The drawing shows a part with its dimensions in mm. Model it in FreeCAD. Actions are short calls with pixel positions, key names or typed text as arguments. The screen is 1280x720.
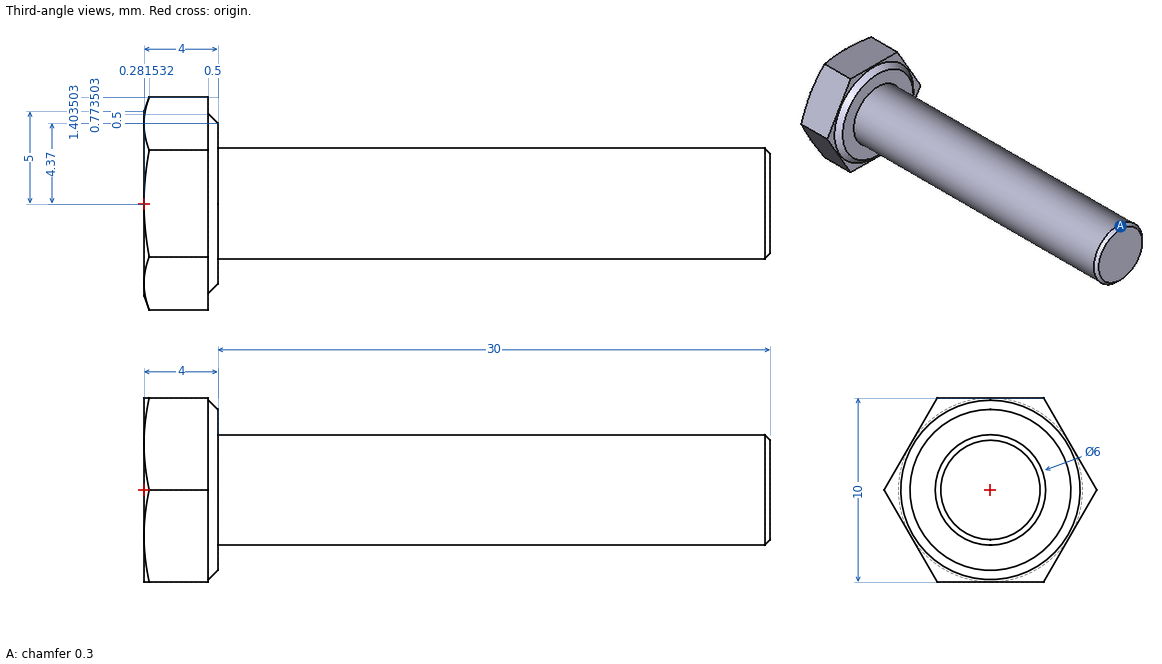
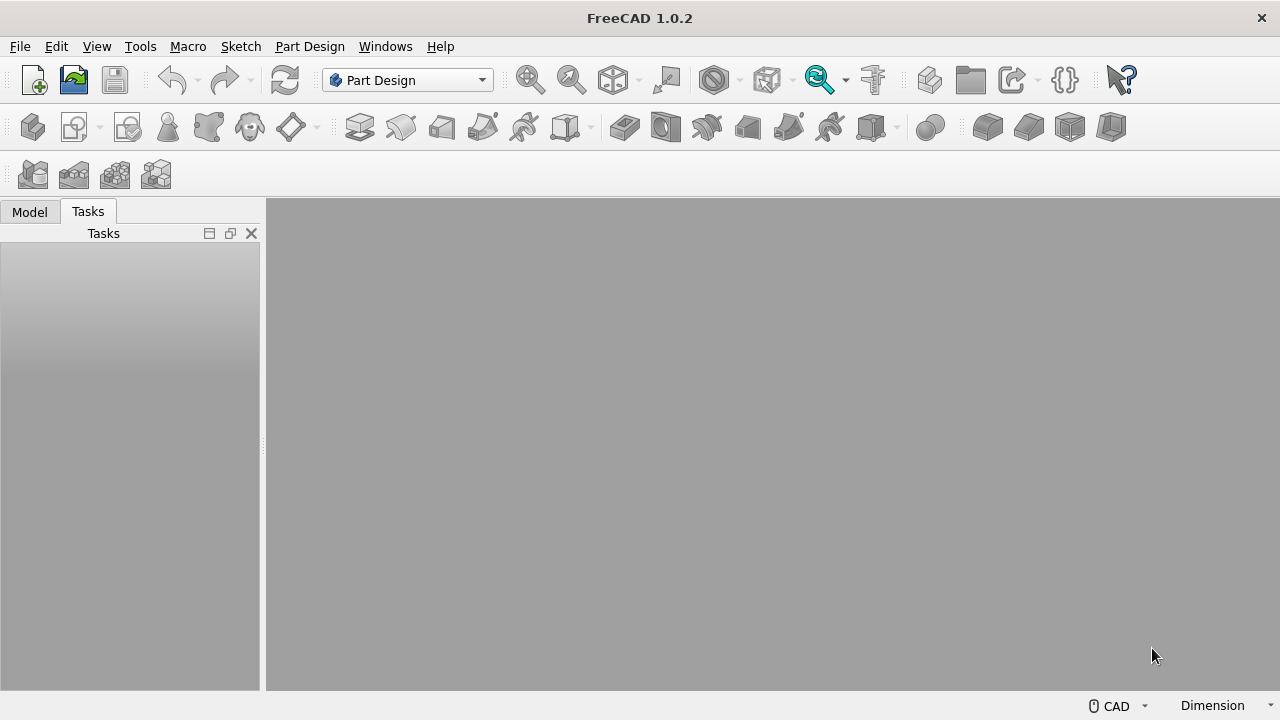
click(33, 80)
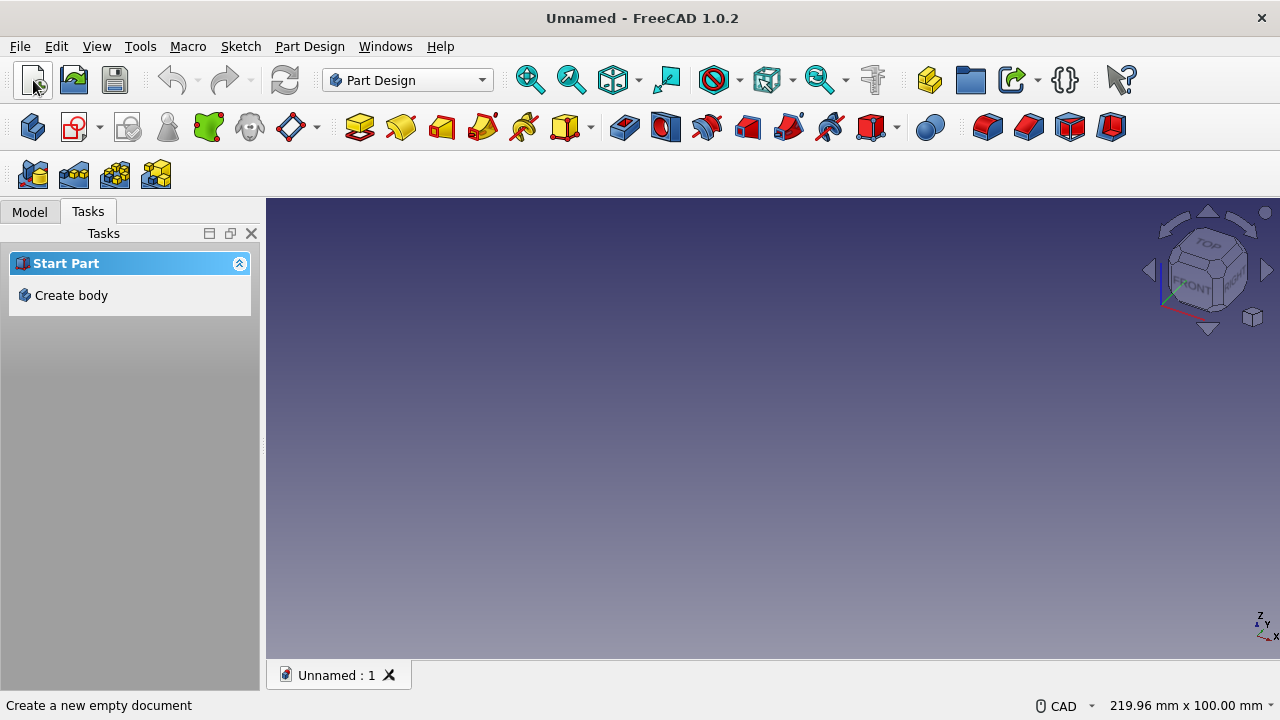
click(74, 128)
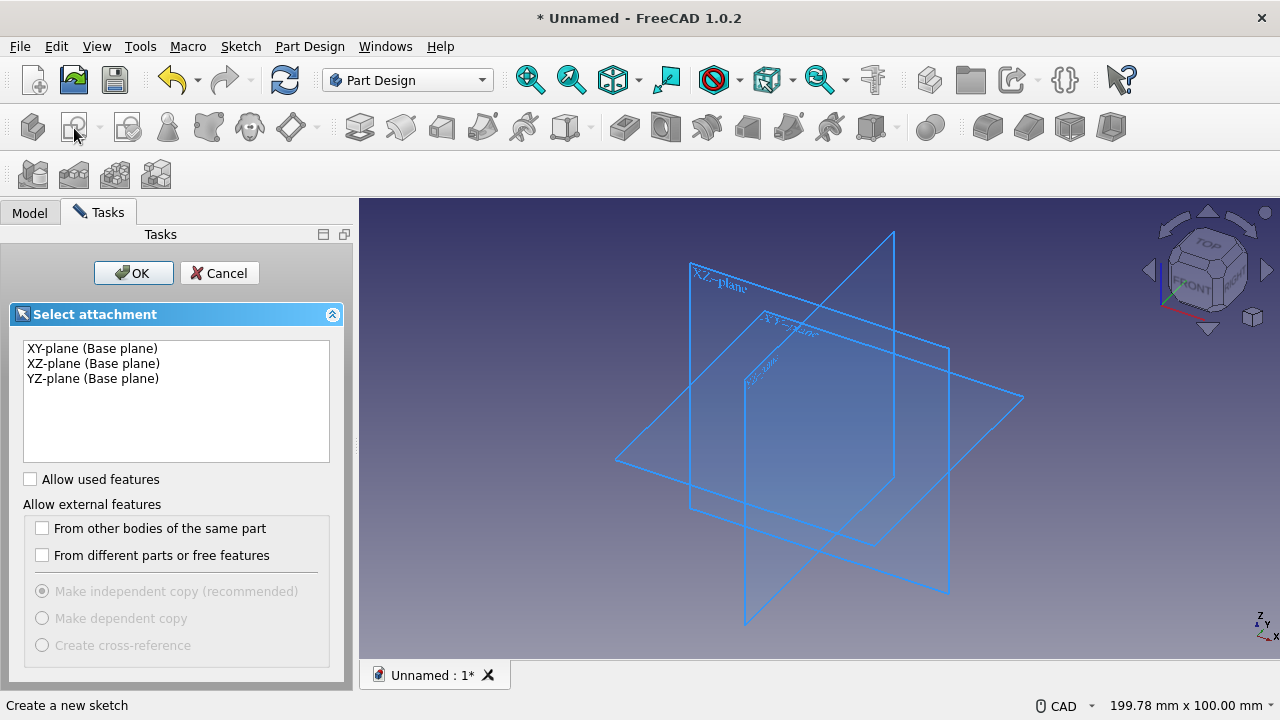
click(84, 378)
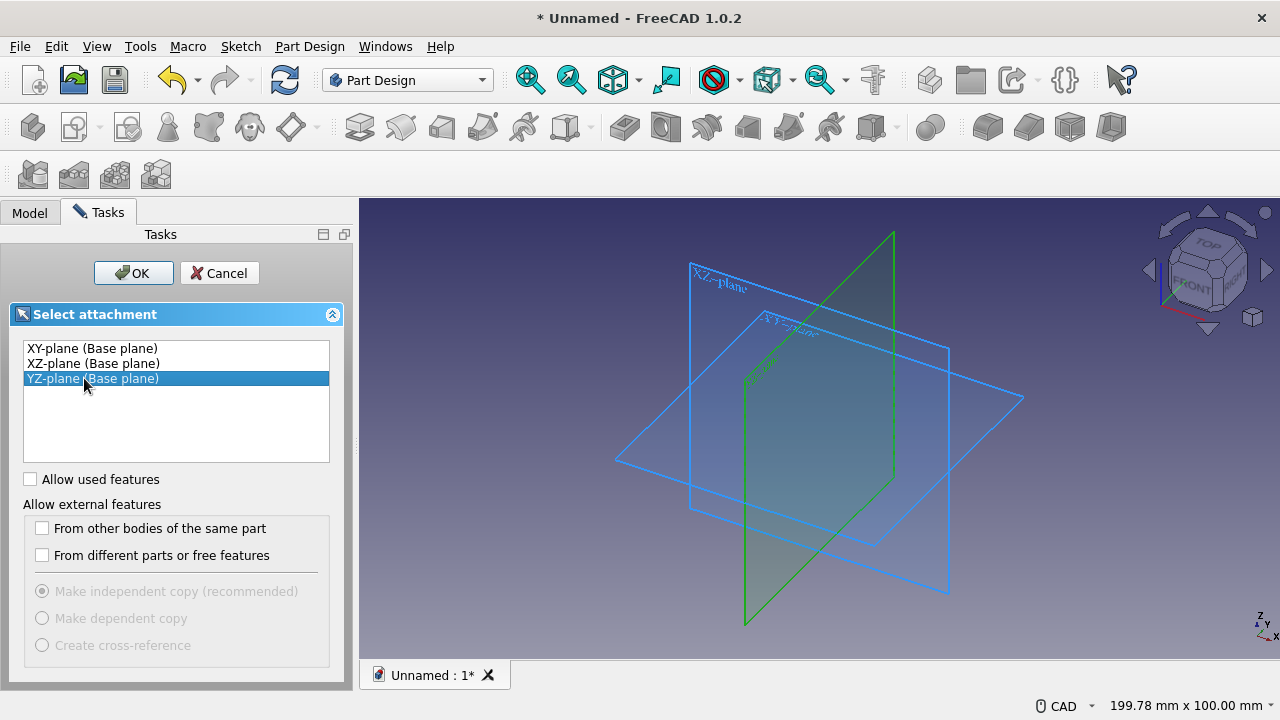
click(134, 273)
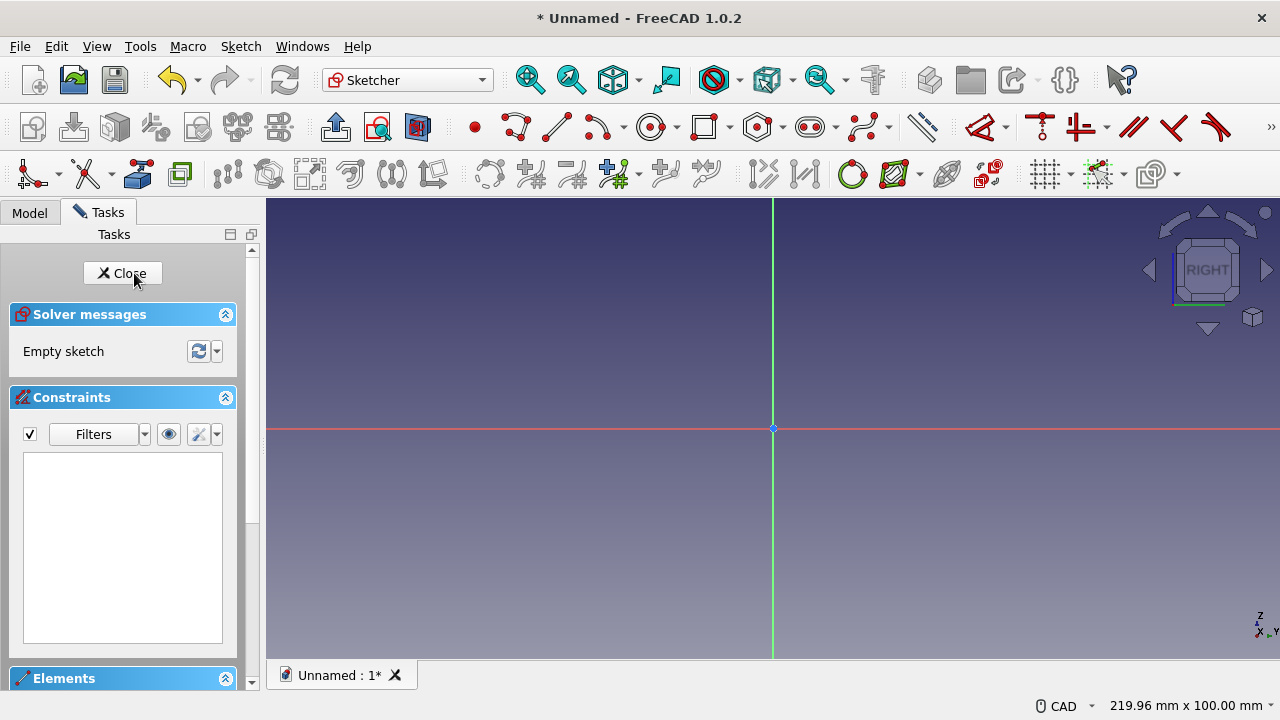
scroll(787, 428, up, 9)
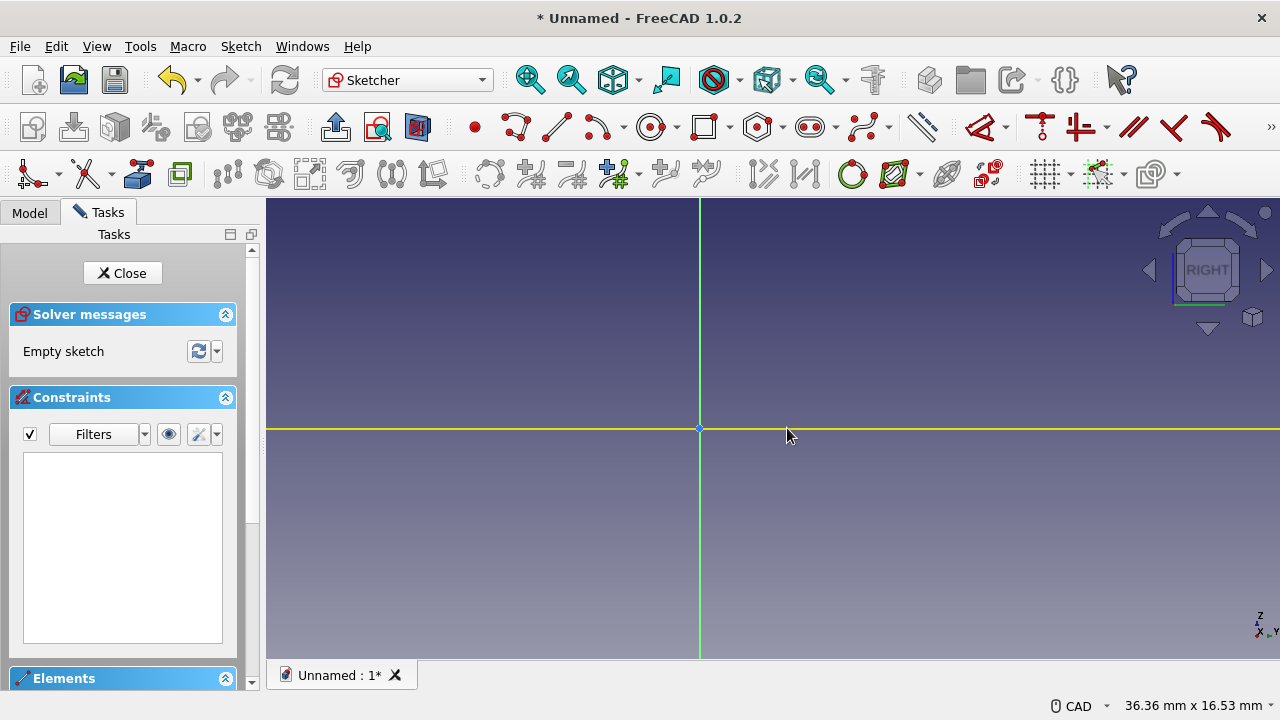
click(756, 128)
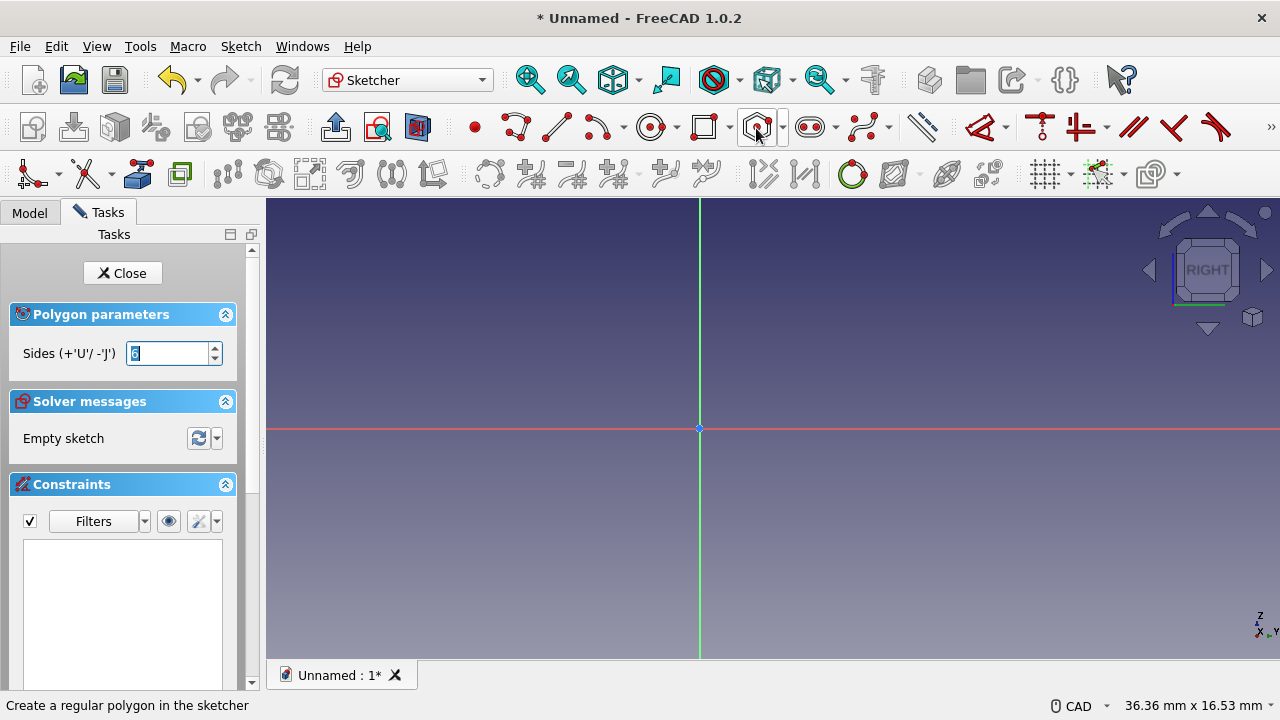
click(700, 428)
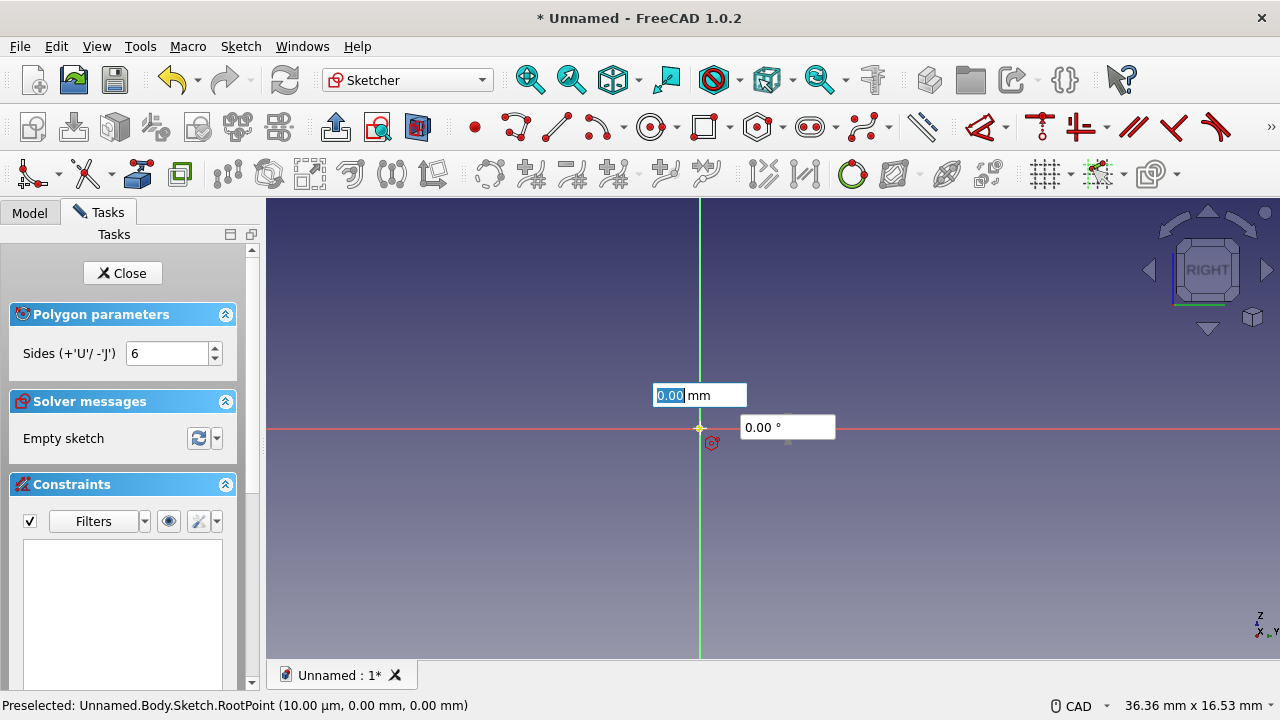
click(539, 428)
right_click(539, 428)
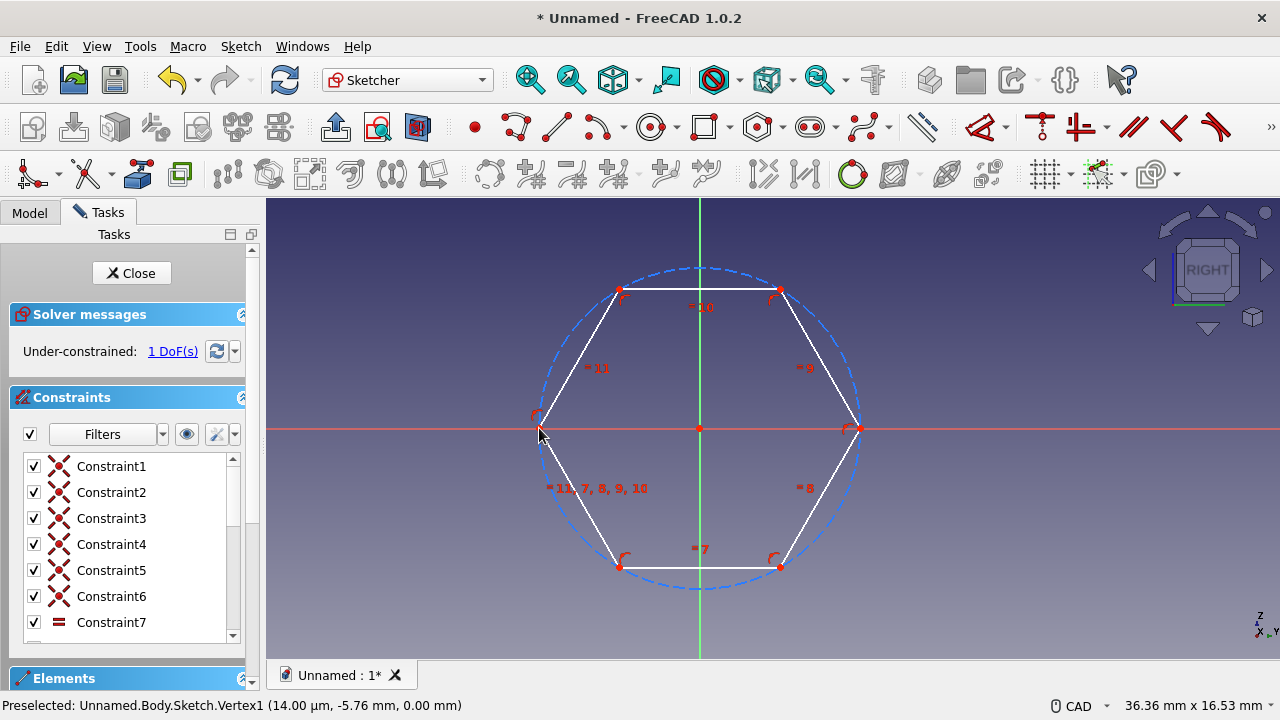
click(980, 128)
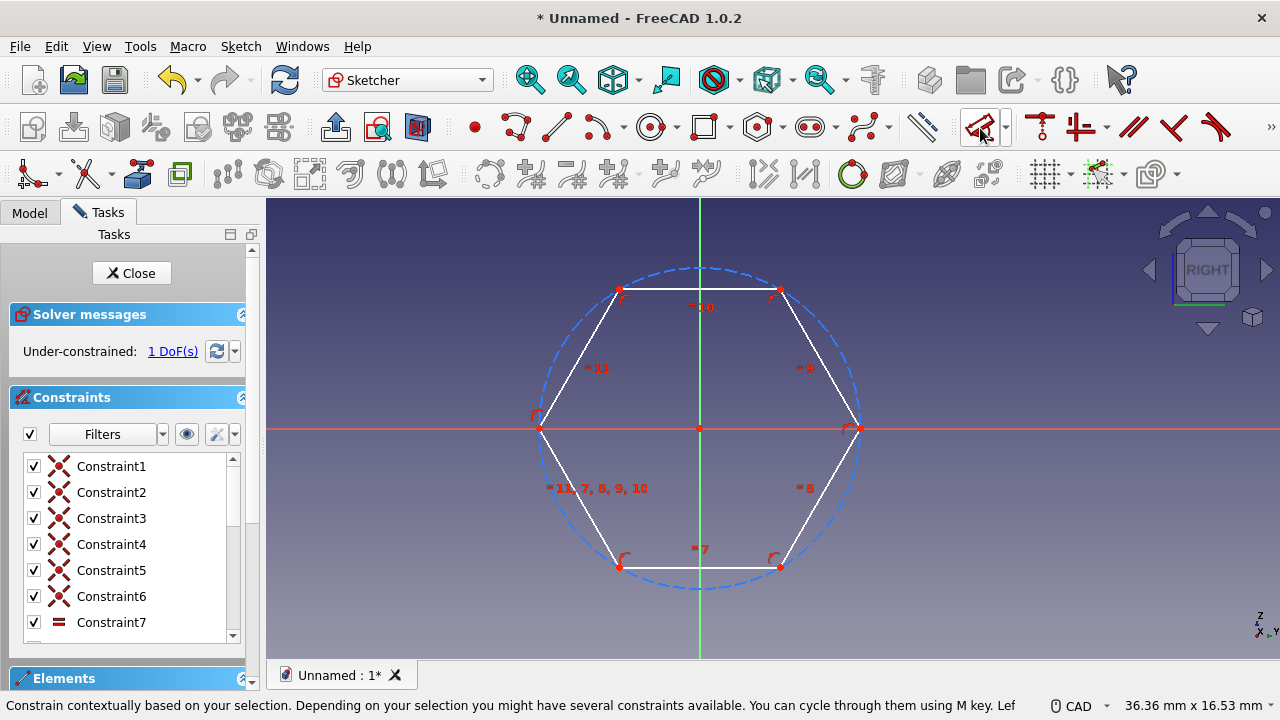
click(619, 568)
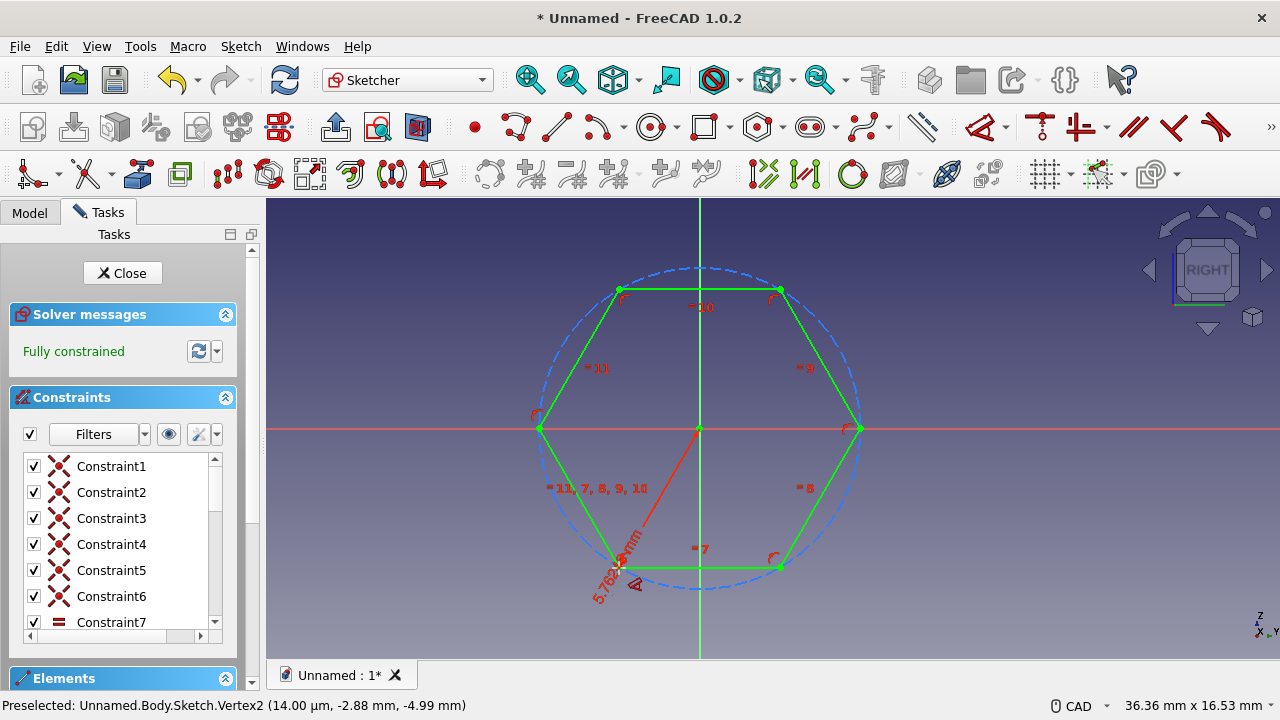
click(780, 289)
click(862, 364)